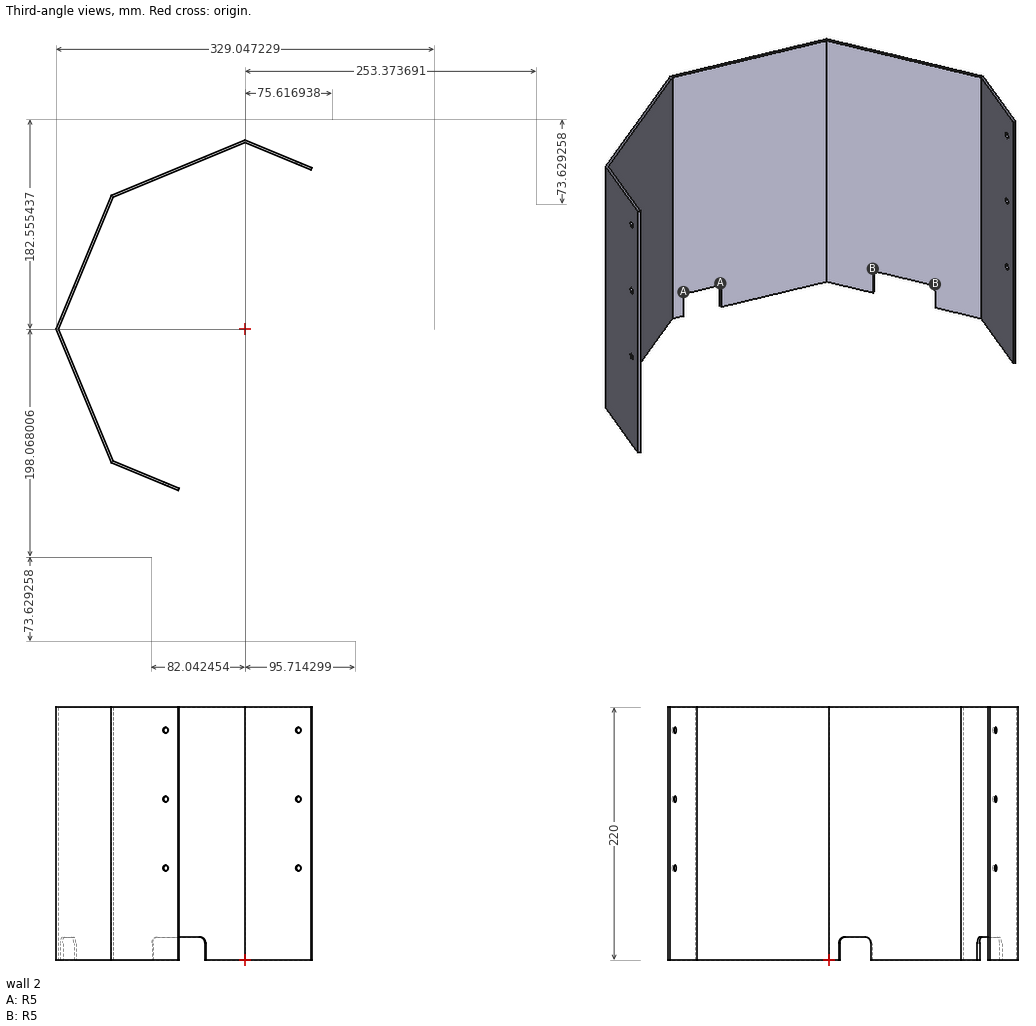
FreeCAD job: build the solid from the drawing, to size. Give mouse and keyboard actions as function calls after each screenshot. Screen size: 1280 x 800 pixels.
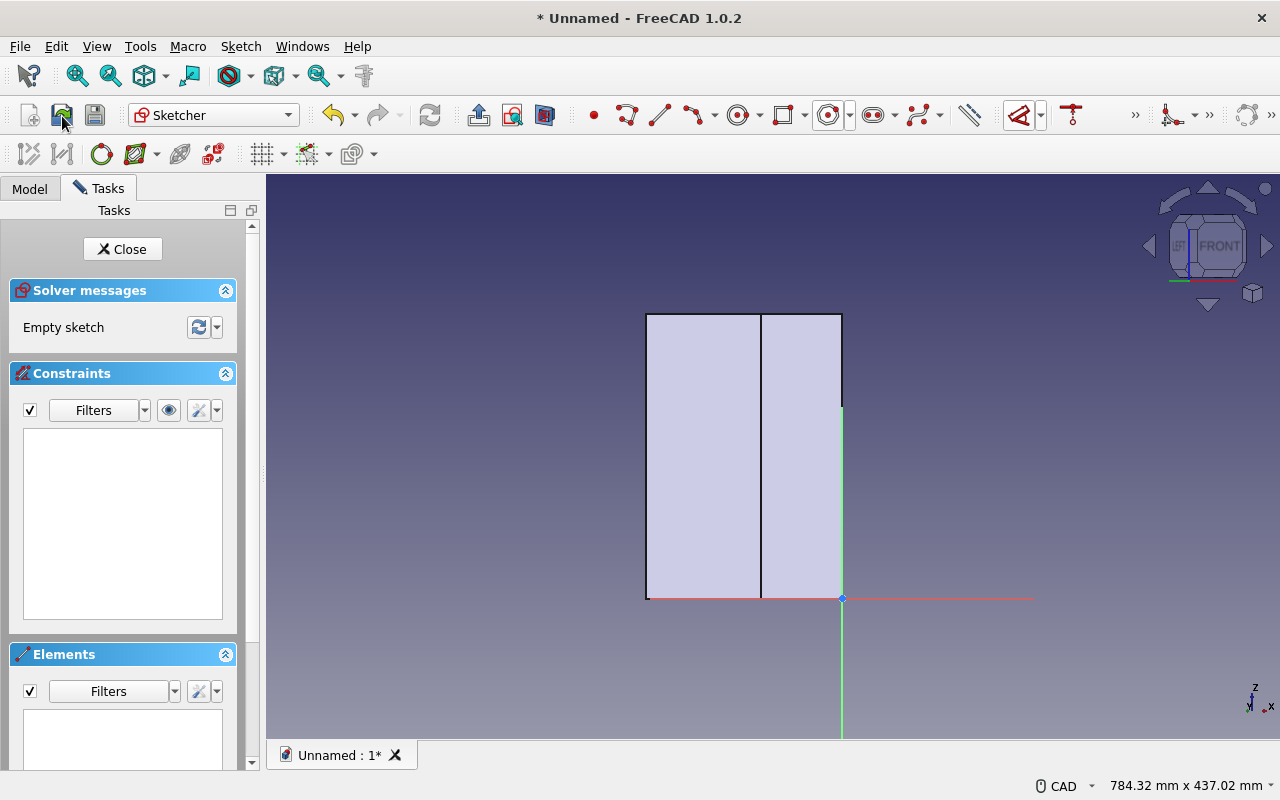
click(545, 116)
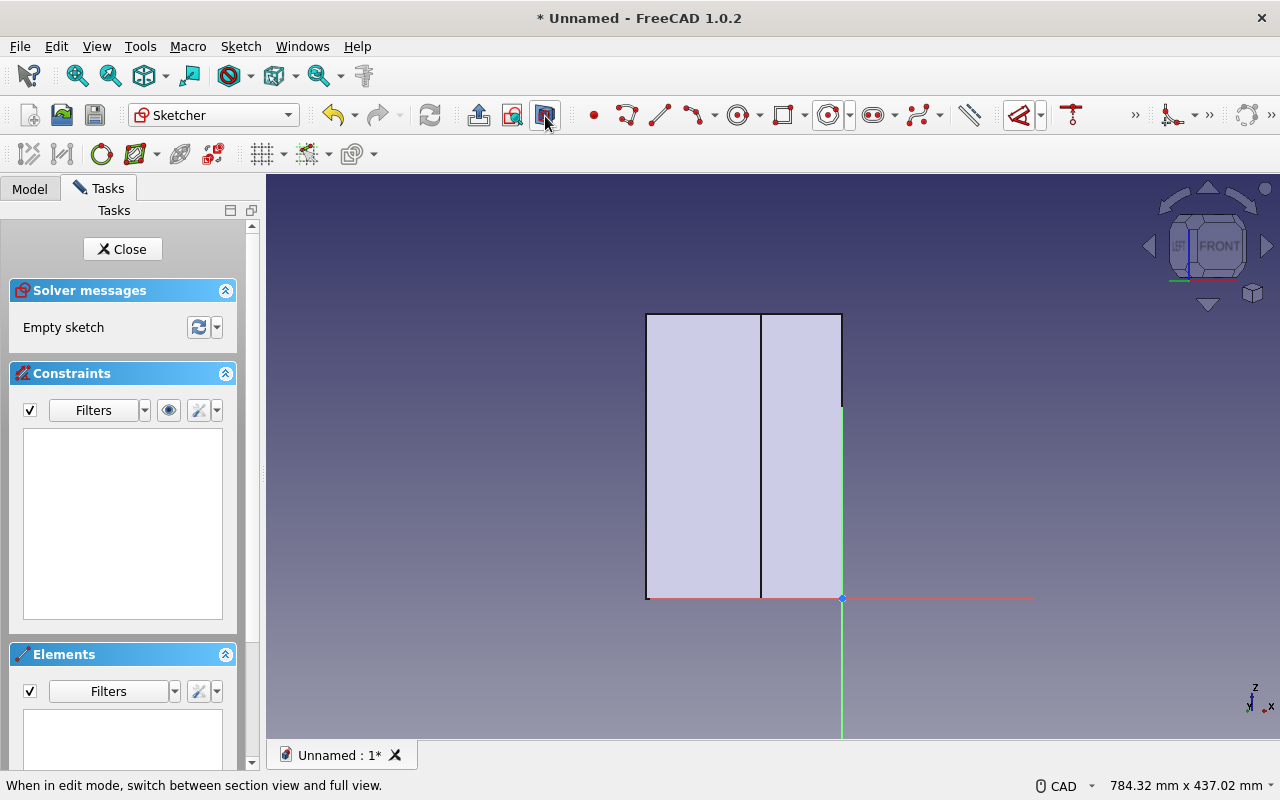
scroll(1095, 491, up, 2)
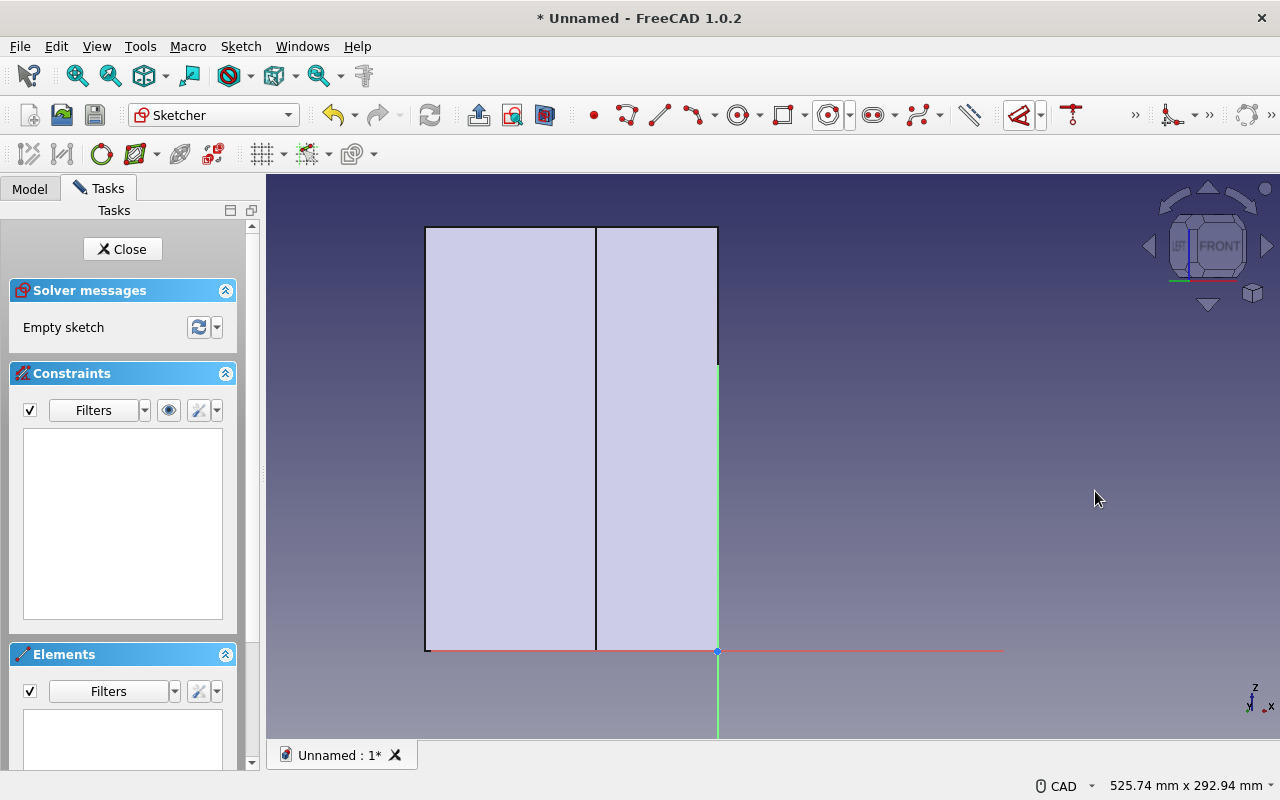
click(738, 116)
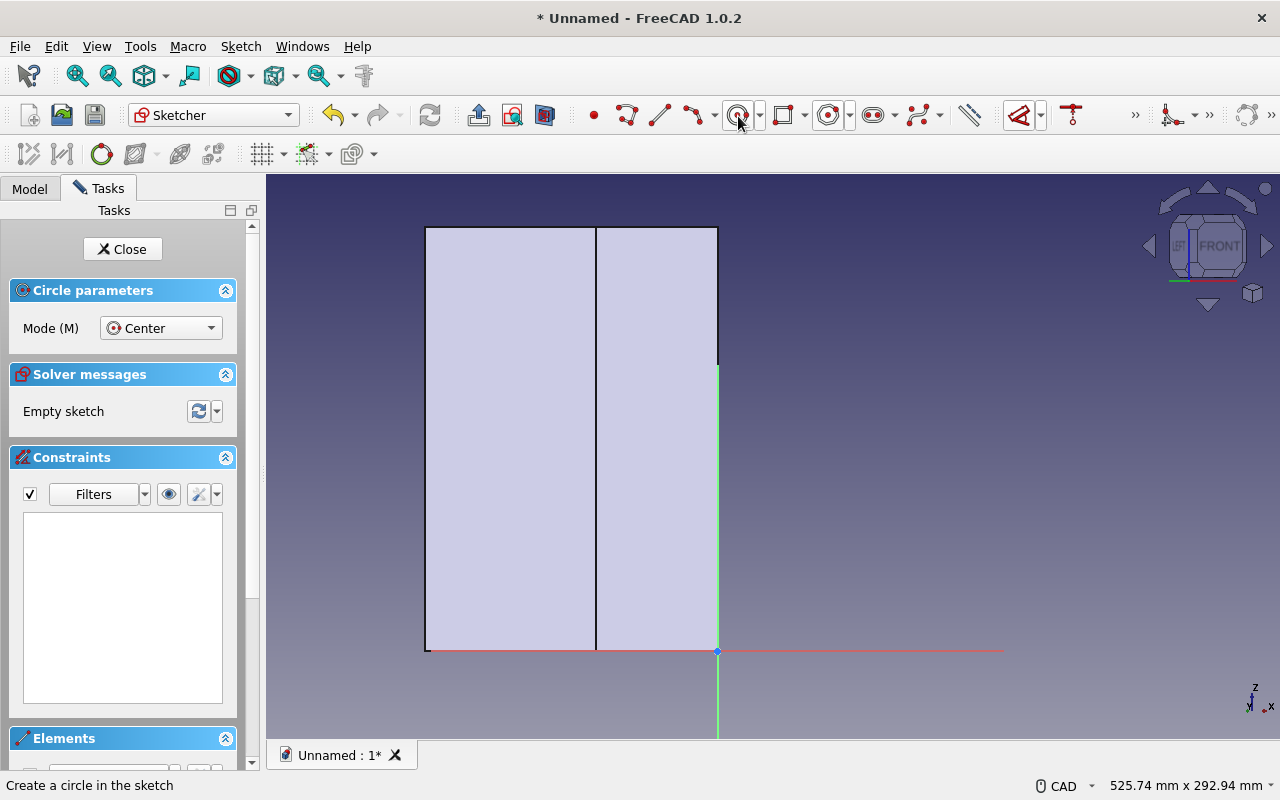
scroll(695, 266, up, 8)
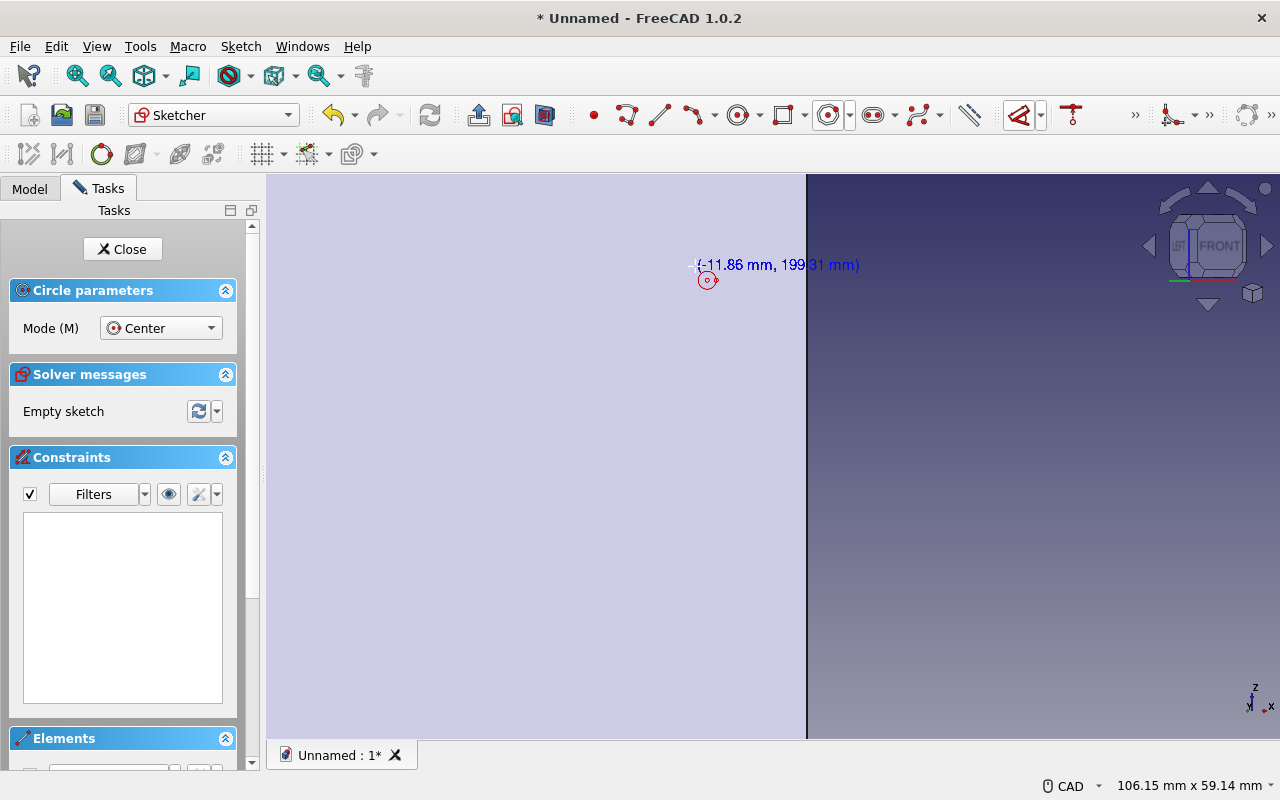
scroll(696, 267, down, 8)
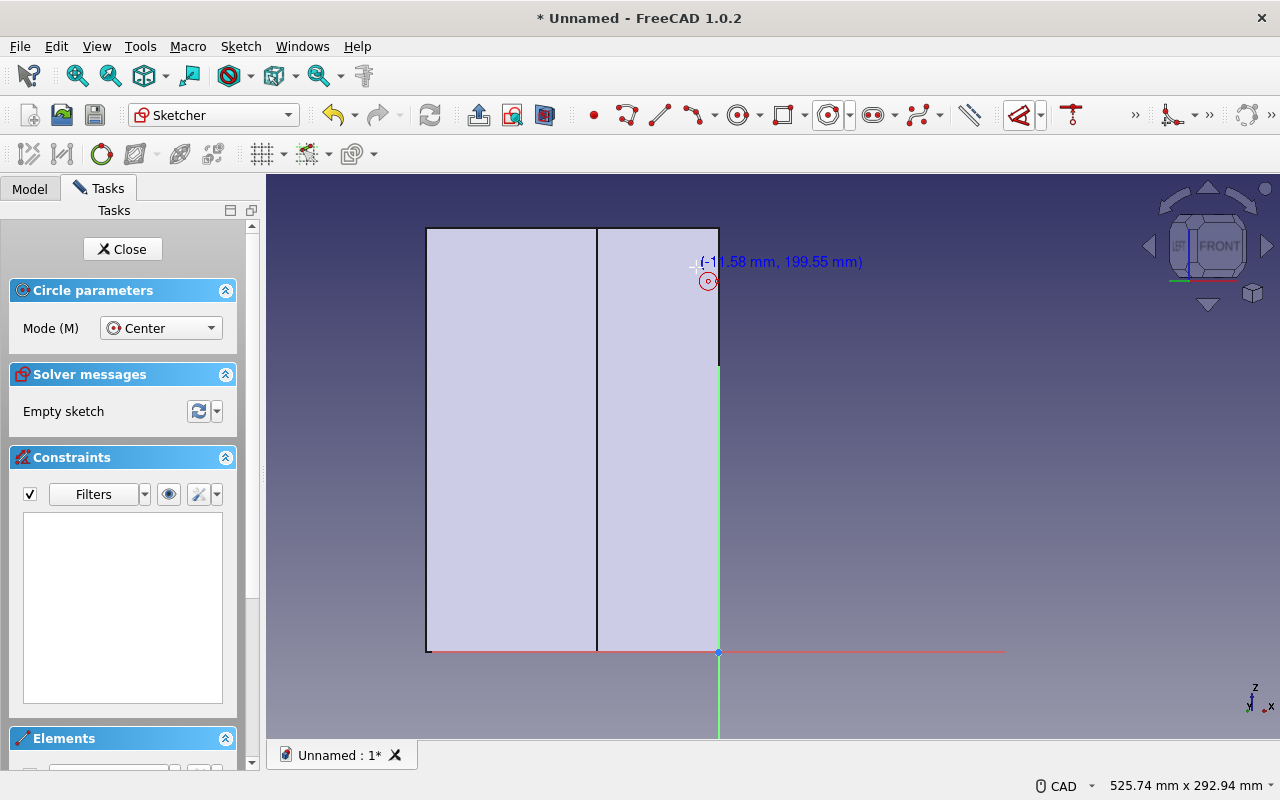
click(696, 266)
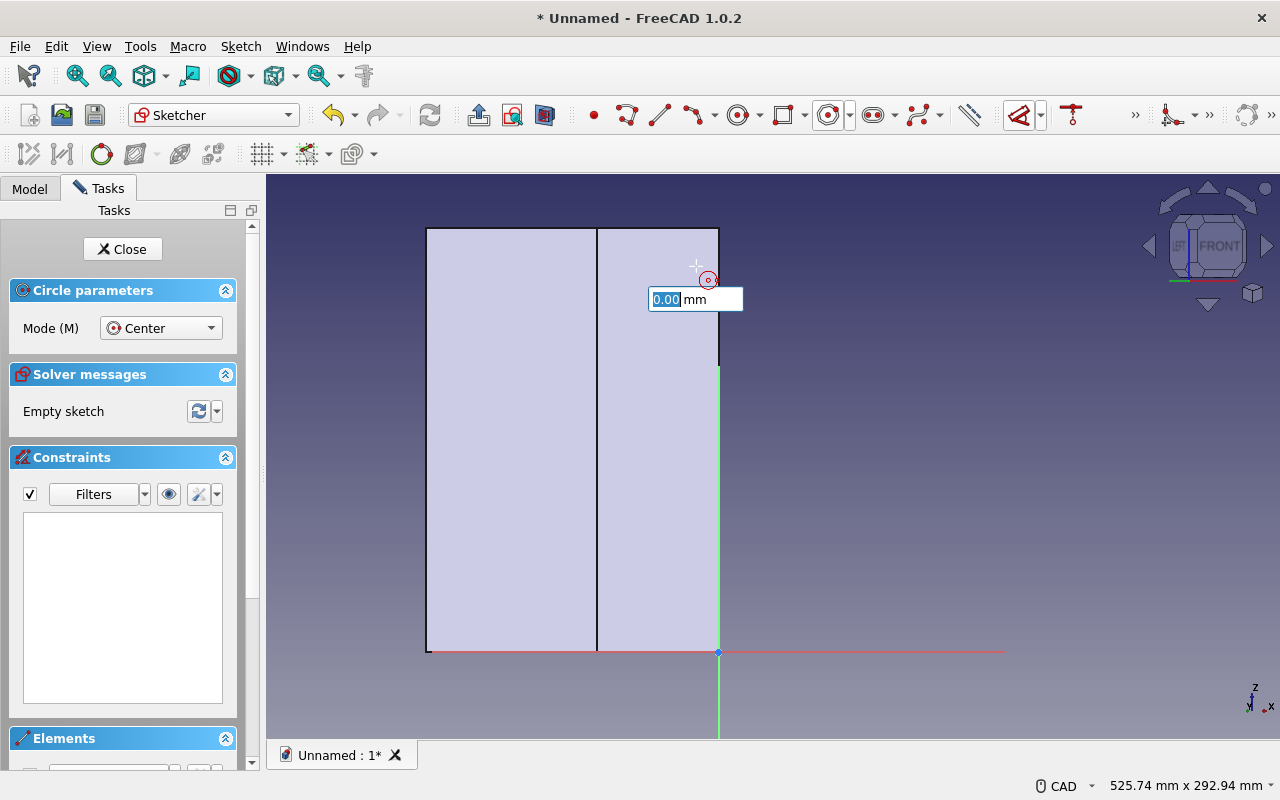
scroll(699, 263, up, 6)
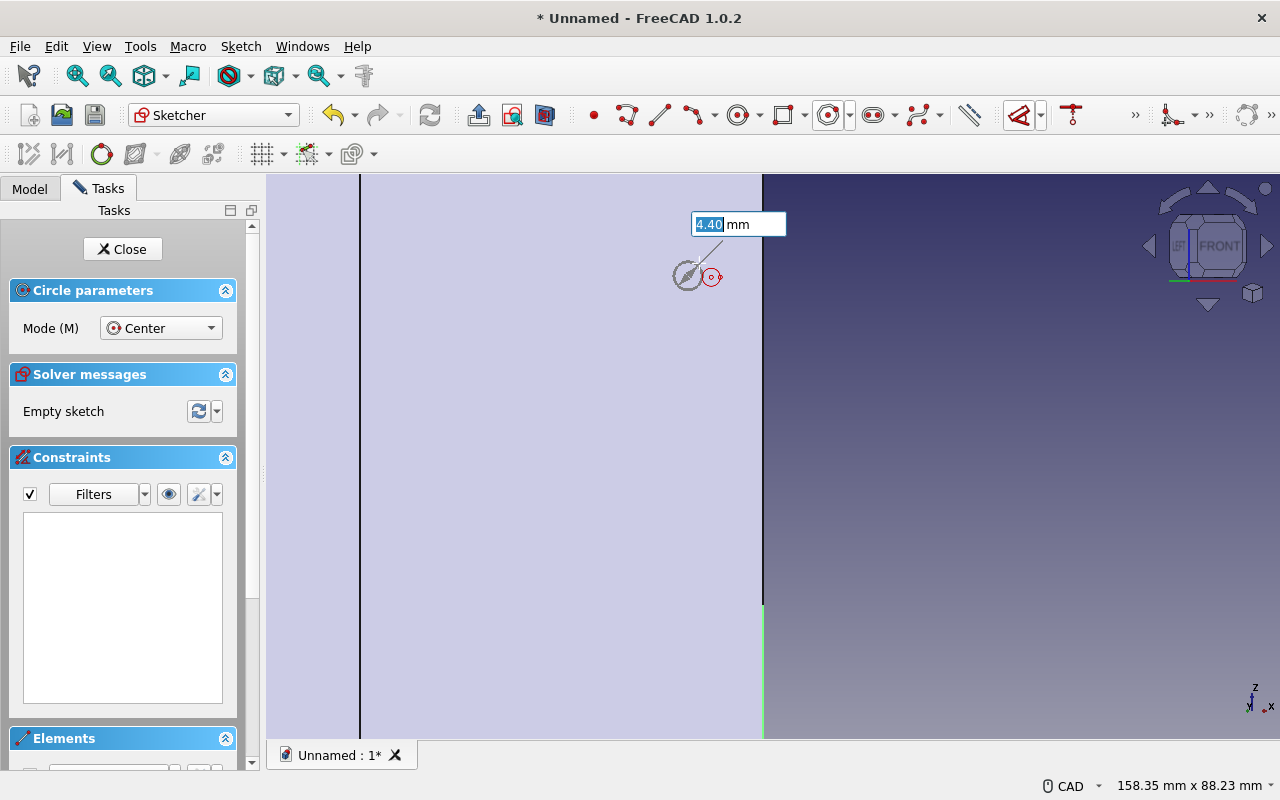
click(698, 263)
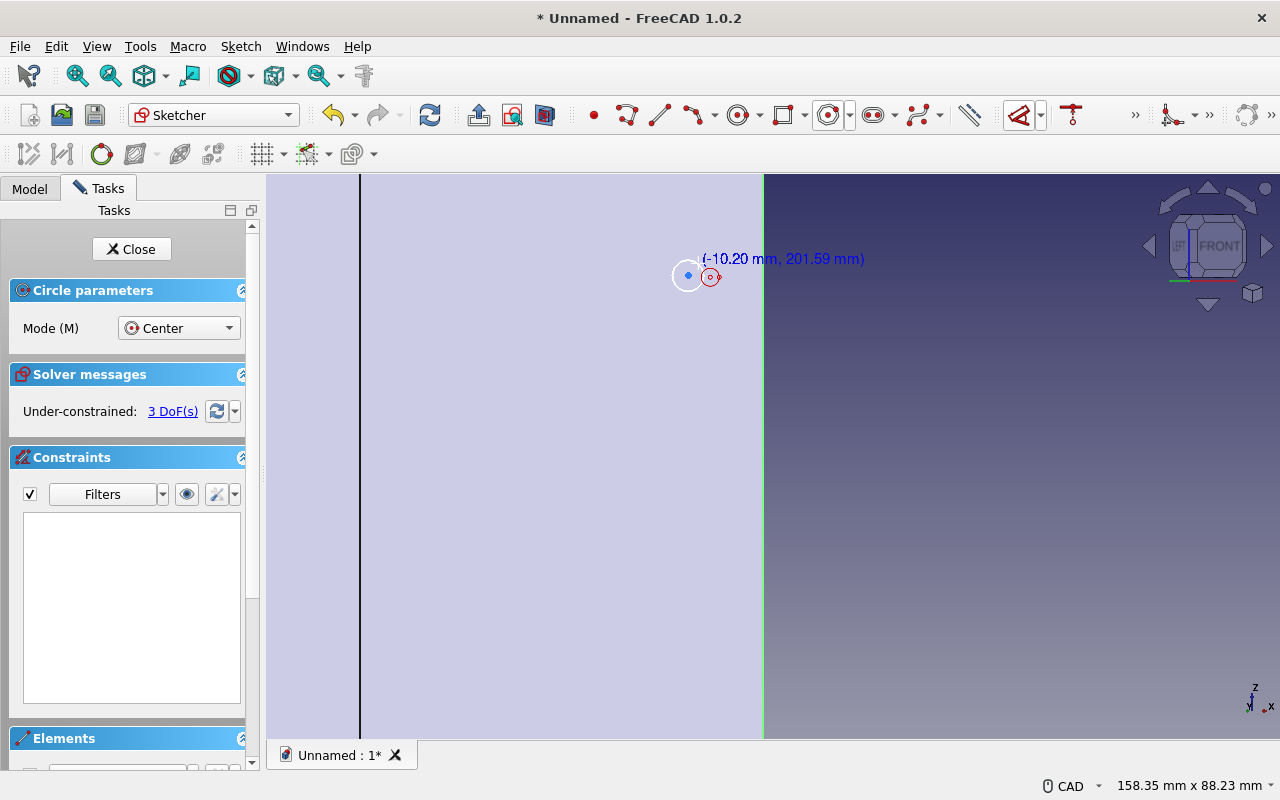
scroll(686, 658, up, 2)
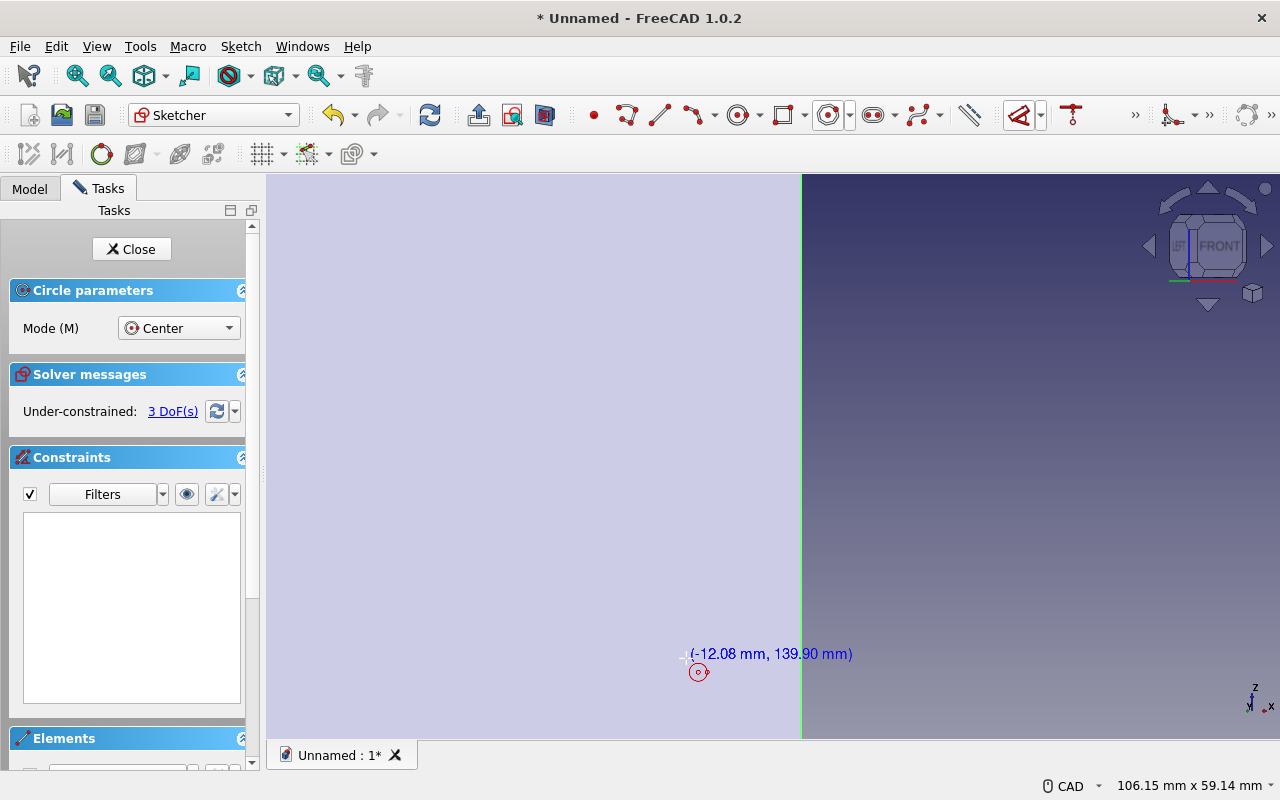
scroll(698, 312, down, 8)